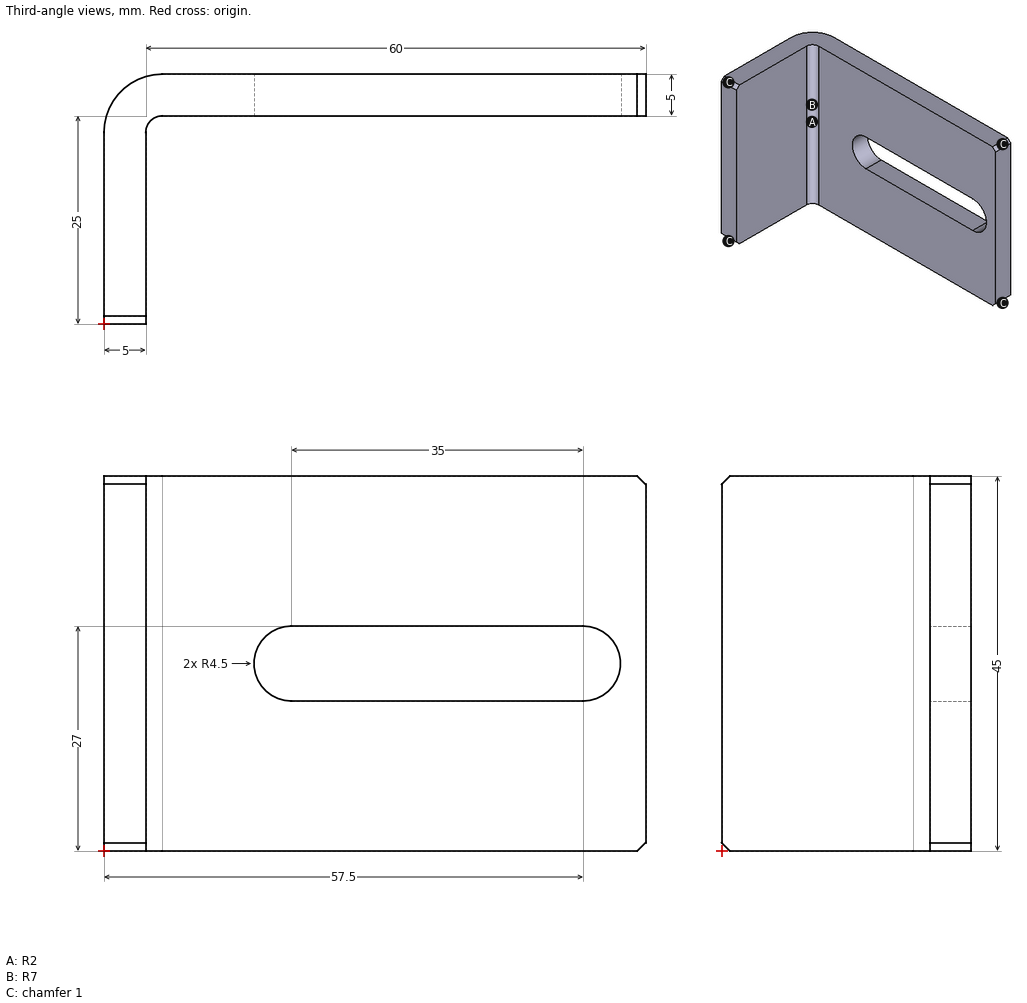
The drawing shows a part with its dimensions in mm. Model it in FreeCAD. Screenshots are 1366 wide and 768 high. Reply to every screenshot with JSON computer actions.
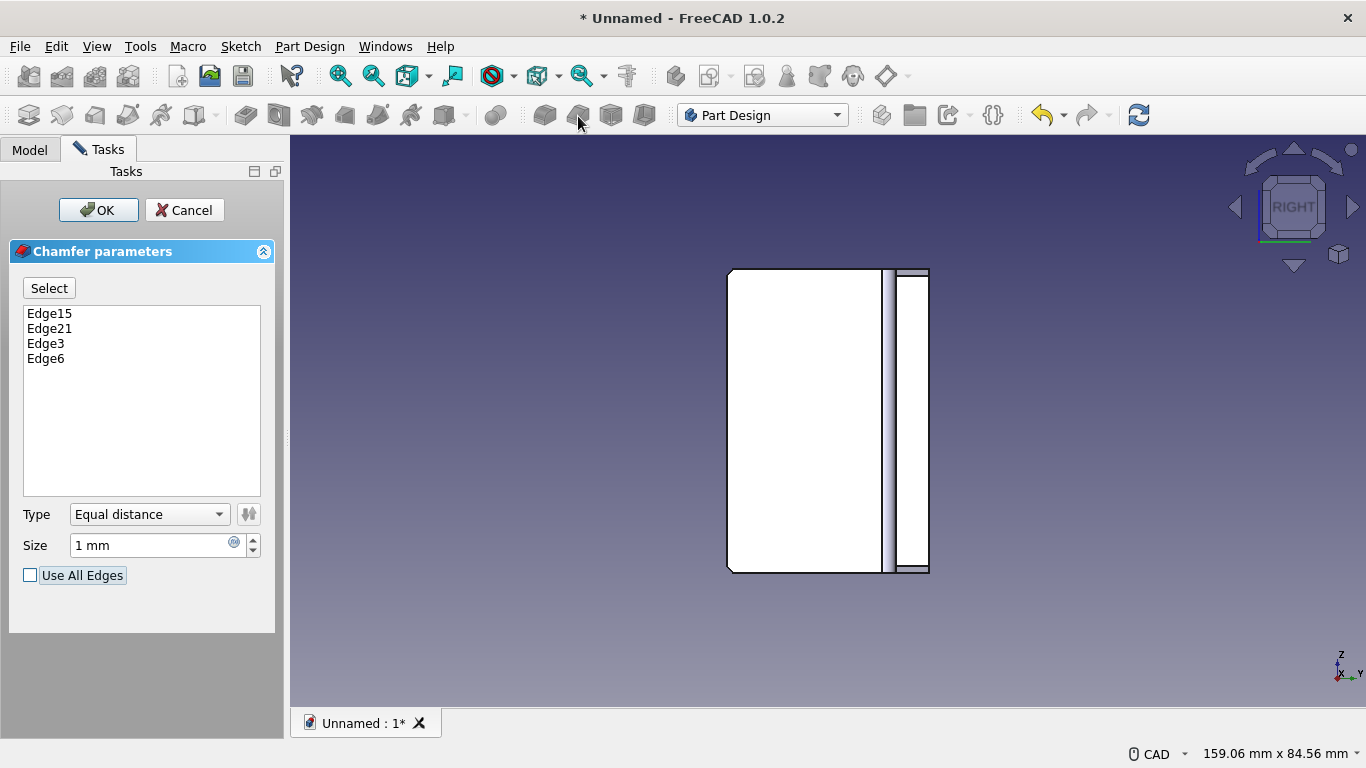
{"action": "left_click", "coordinate": [99, 210]}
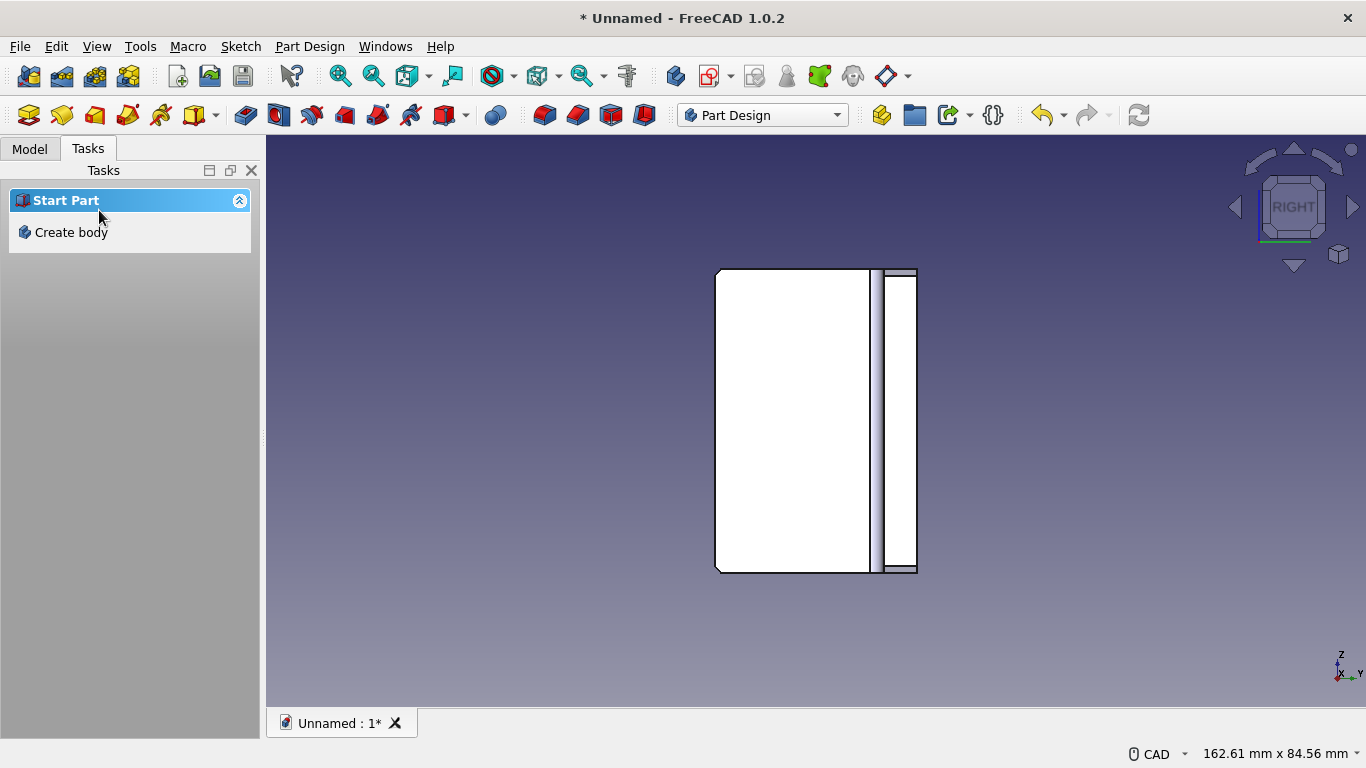
{"action": "key", "text": "4"}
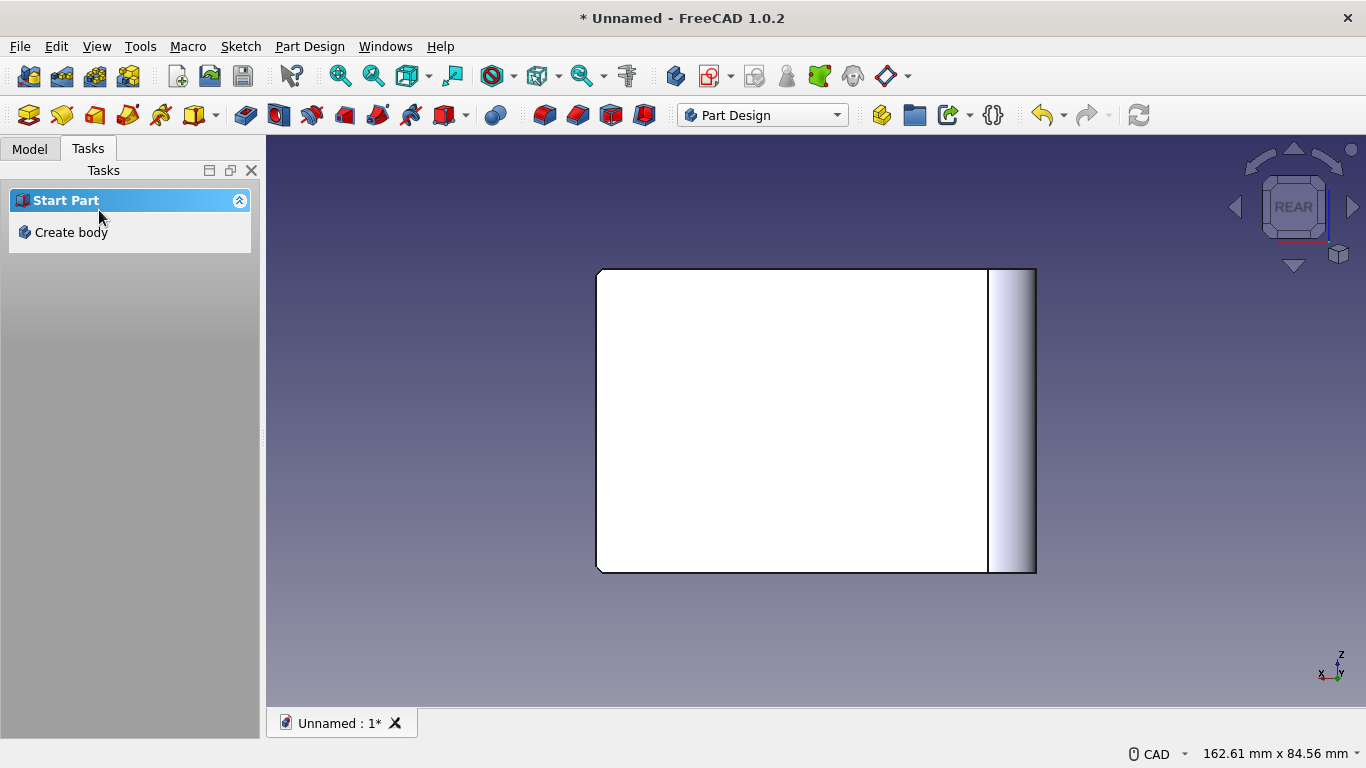
{"action": "left_click", "coordinate": [792, 420]}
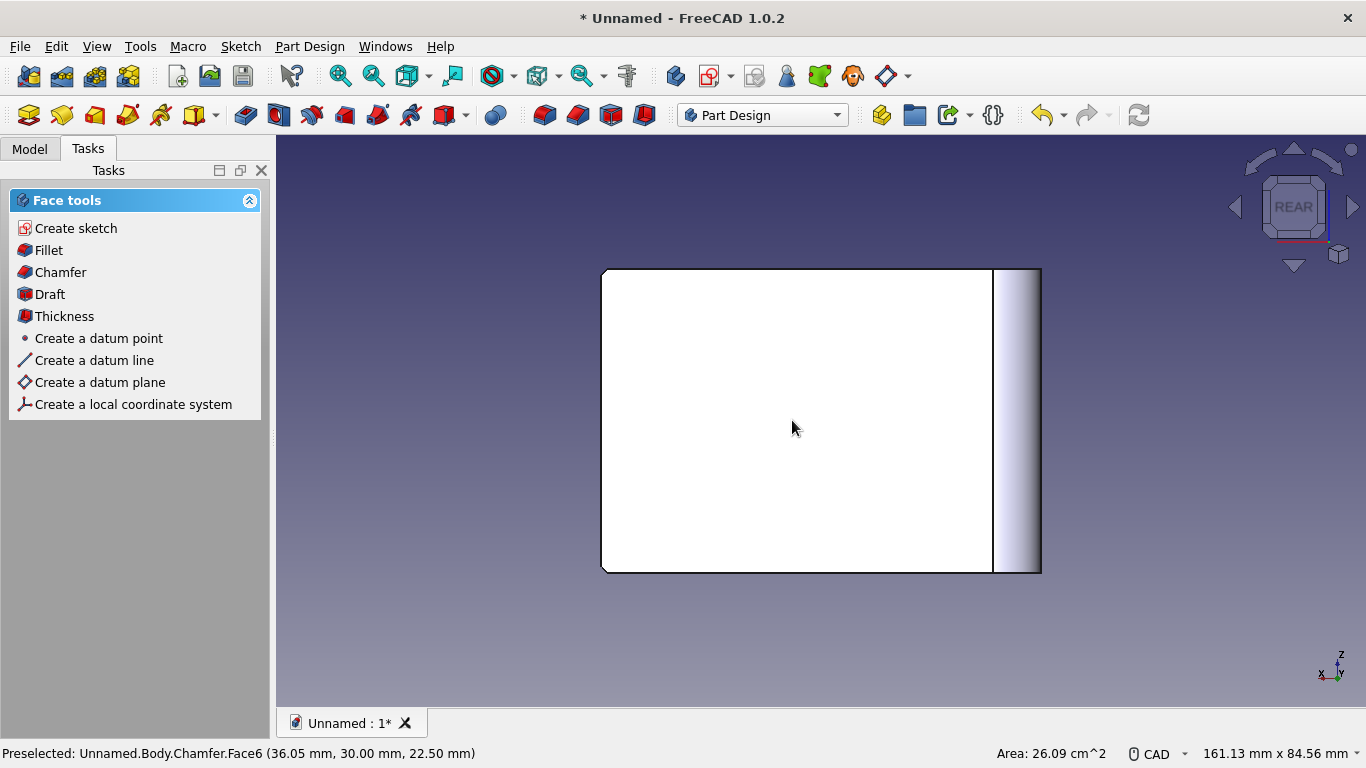
{"action": "left_click", "coordinate": [708, 76]}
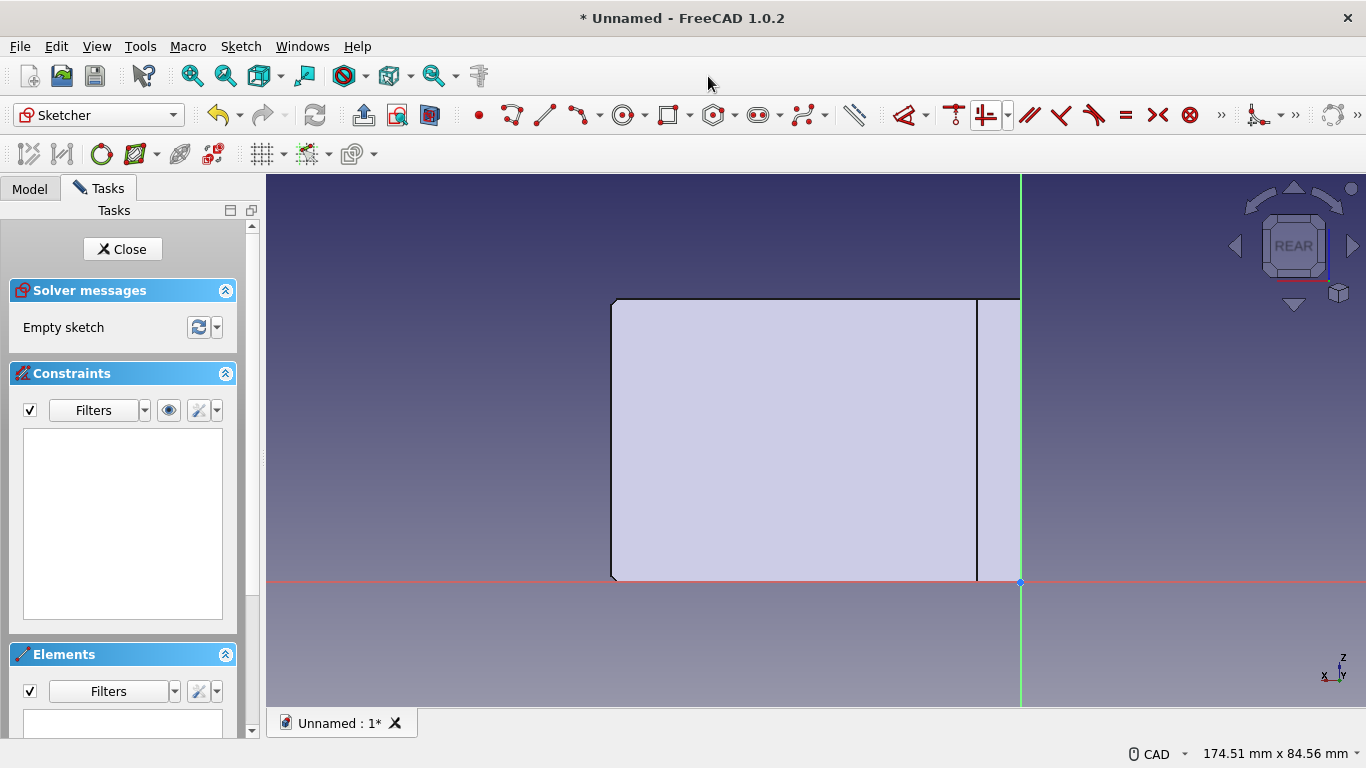
{"action": "scroll", "coordinate": [984, 613], "scroll_direction": "up", "scroll_amount": 2}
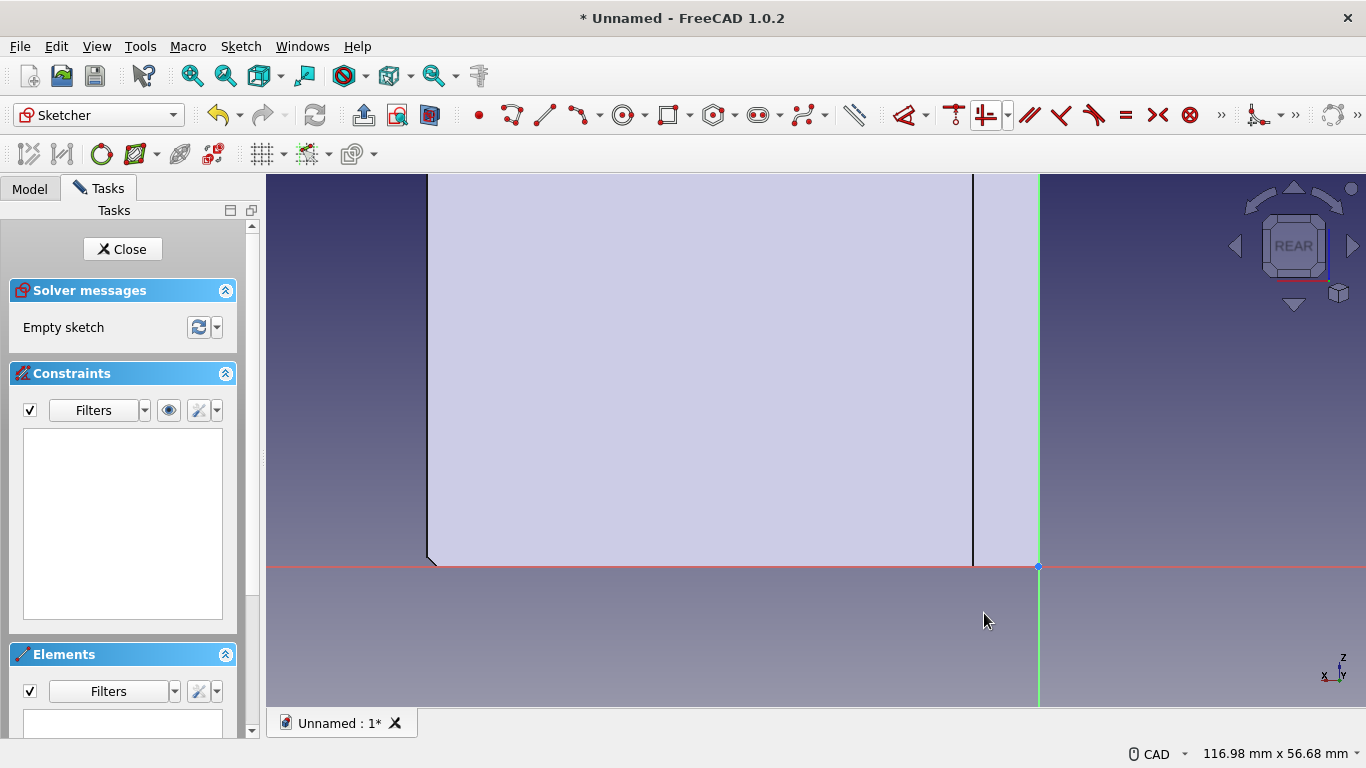
{"action": "key", "text": "g s"}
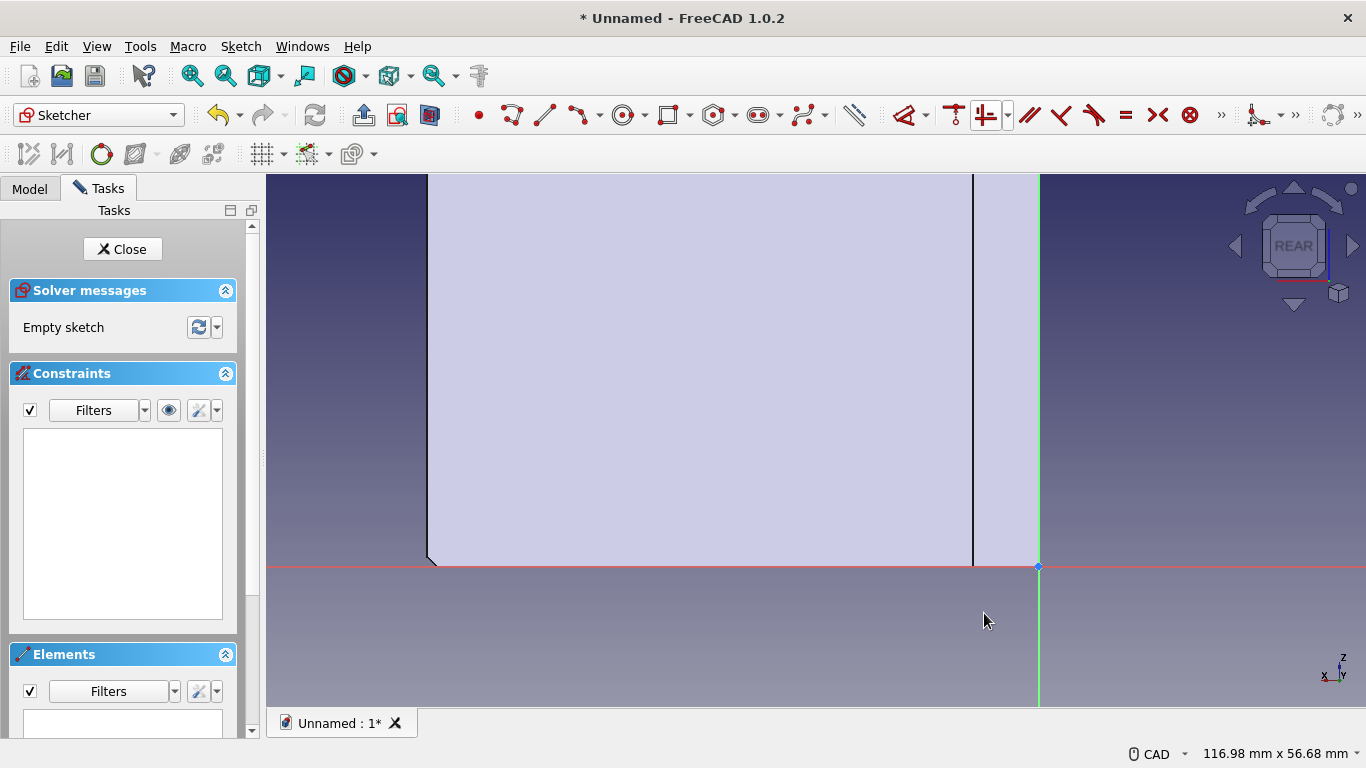
{"action": "left_click", "coordinate": [498, 355]}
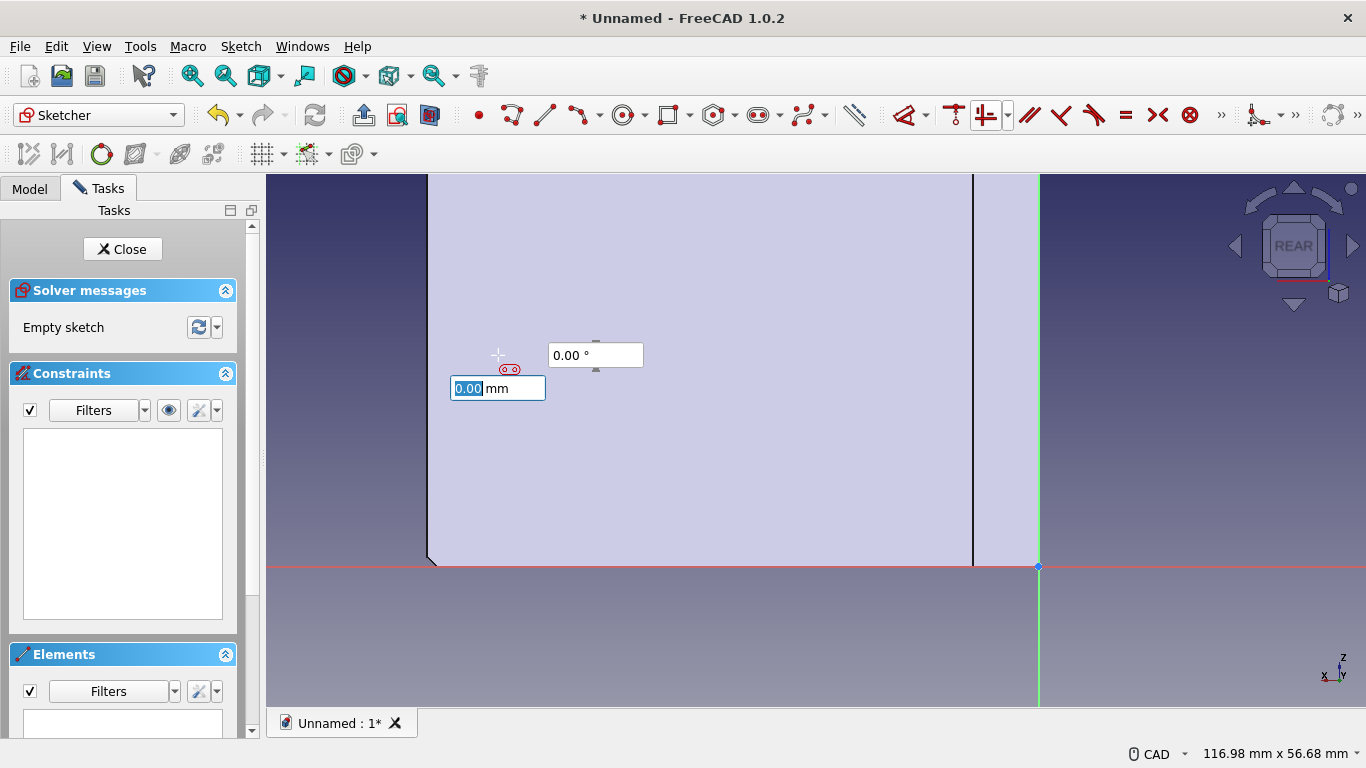
{"action": "left_click", "coordinate": [827, 355]}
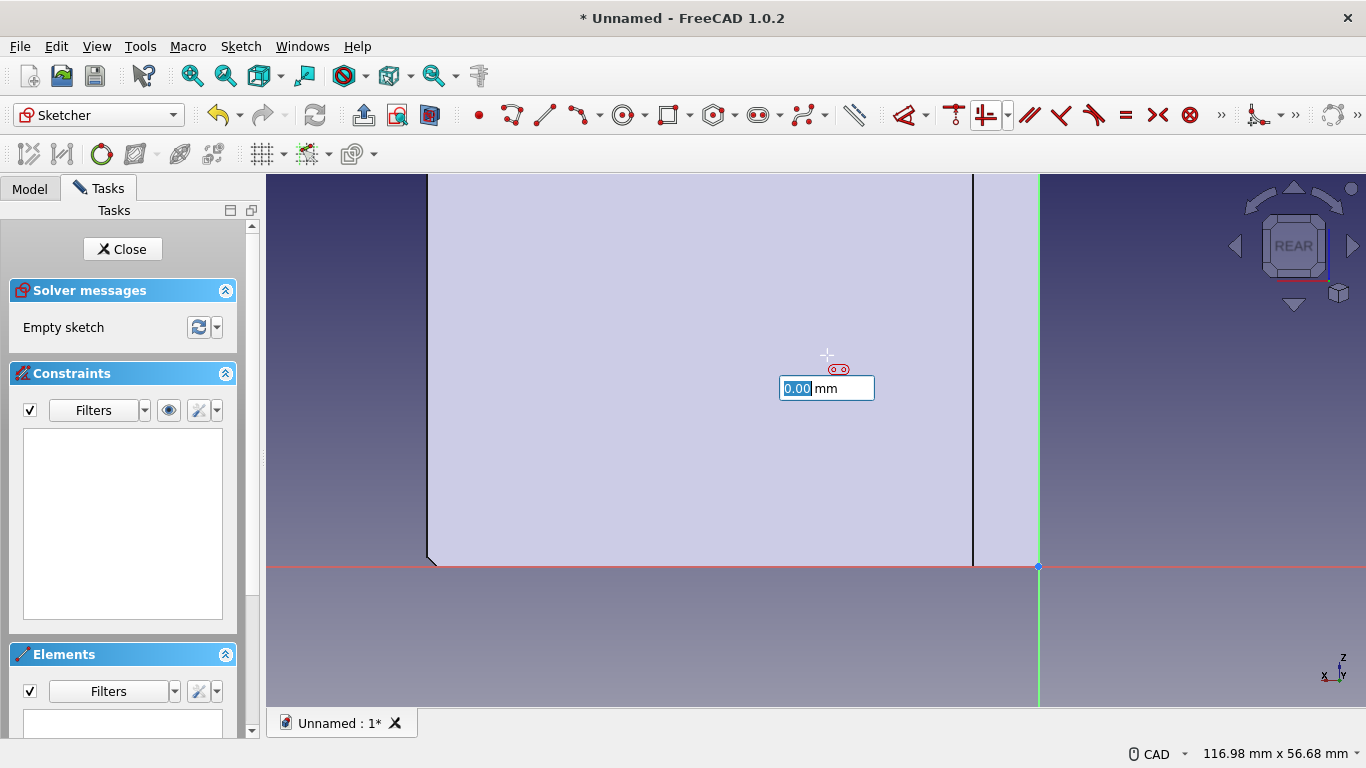
{"action": "left_click", "coordinate": [663, 398]}
{"action": "key", "text": "Escape"}